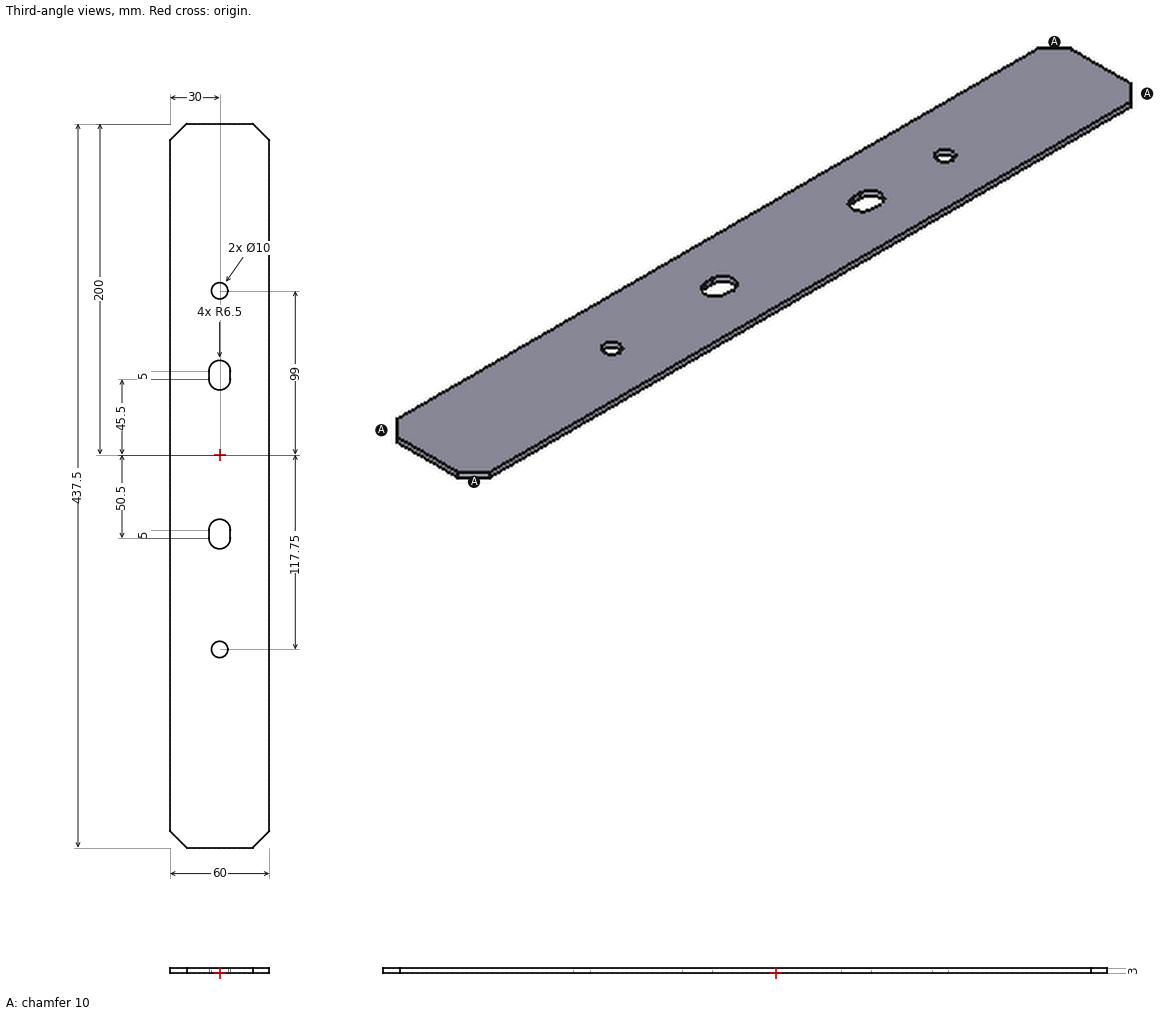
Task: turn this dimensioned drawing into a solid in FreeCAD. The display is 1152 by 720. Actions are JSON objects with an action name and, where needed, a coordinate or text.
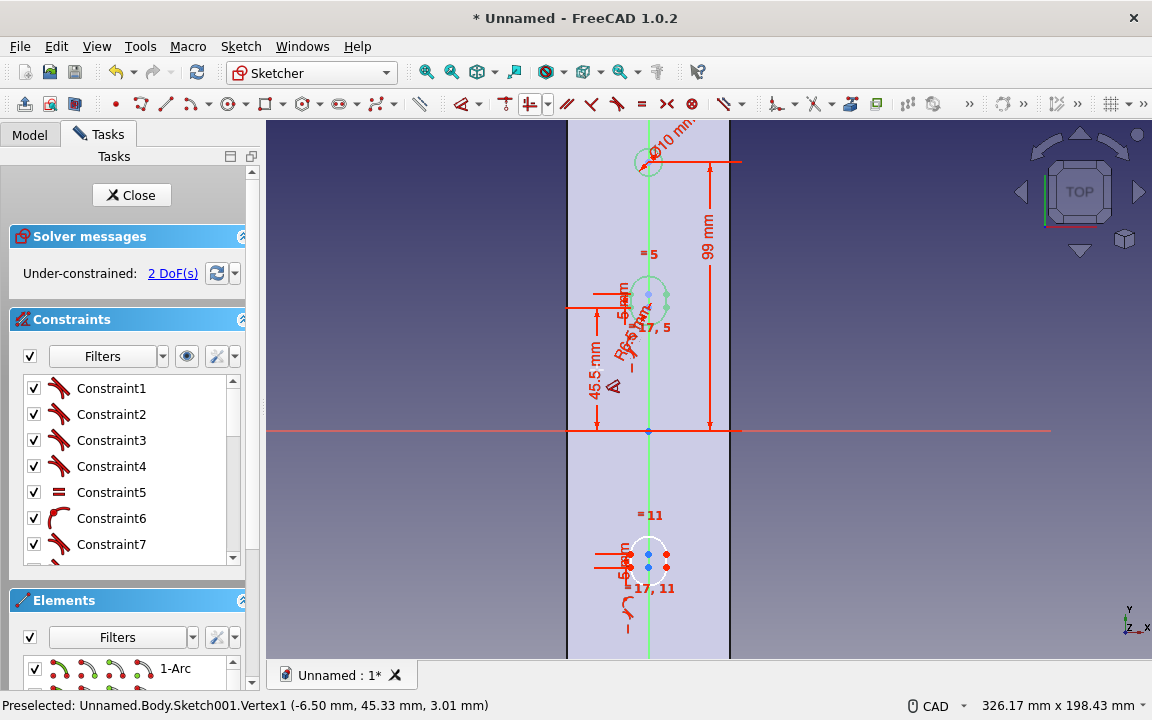
{"action": "left_click", "coordinate": [631, 568]}
{"action": "left_click", "coordinate": [597, 500]}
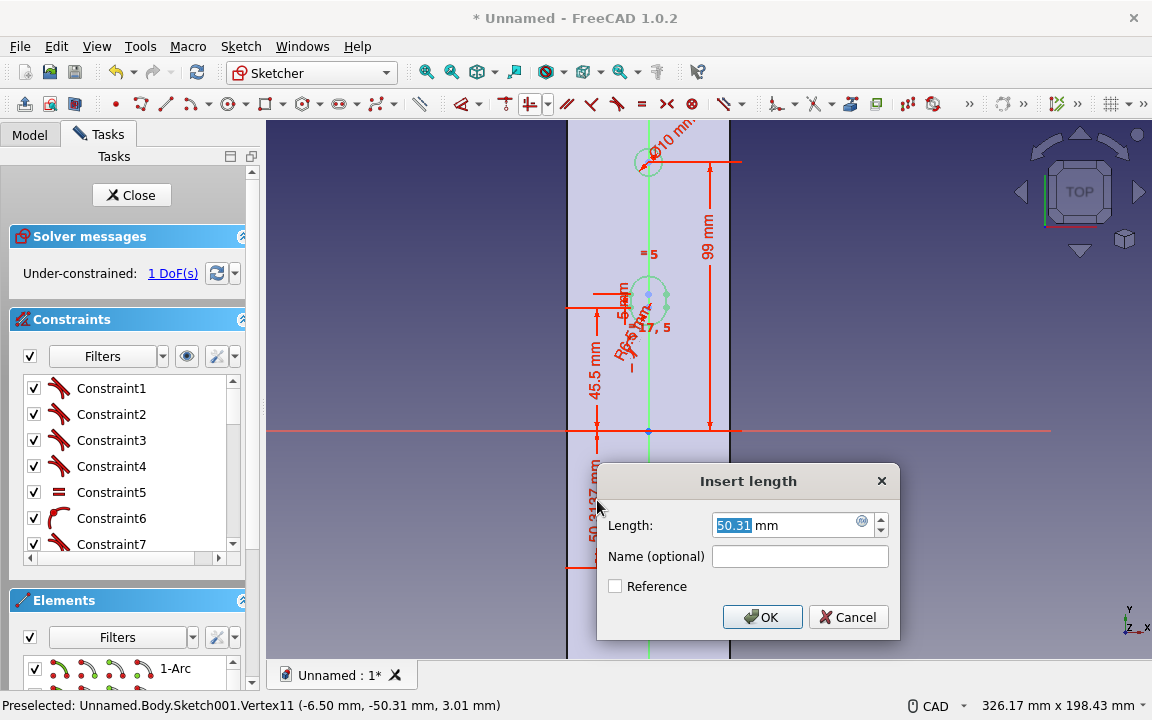
{"action": "type", "text": "50.5"}
{"action": "key", "text": "Return"}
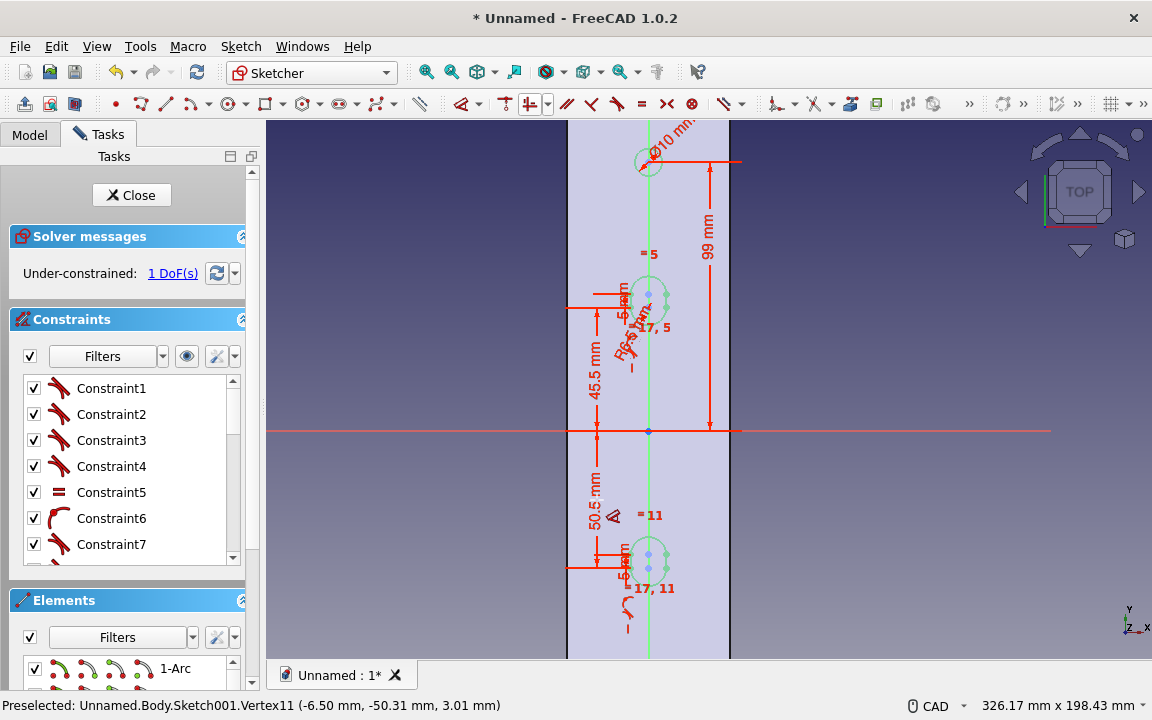
{"action": "scroll", "coordinate": [631, 308], "scroll_direction": "down", "scroll_amount": 3}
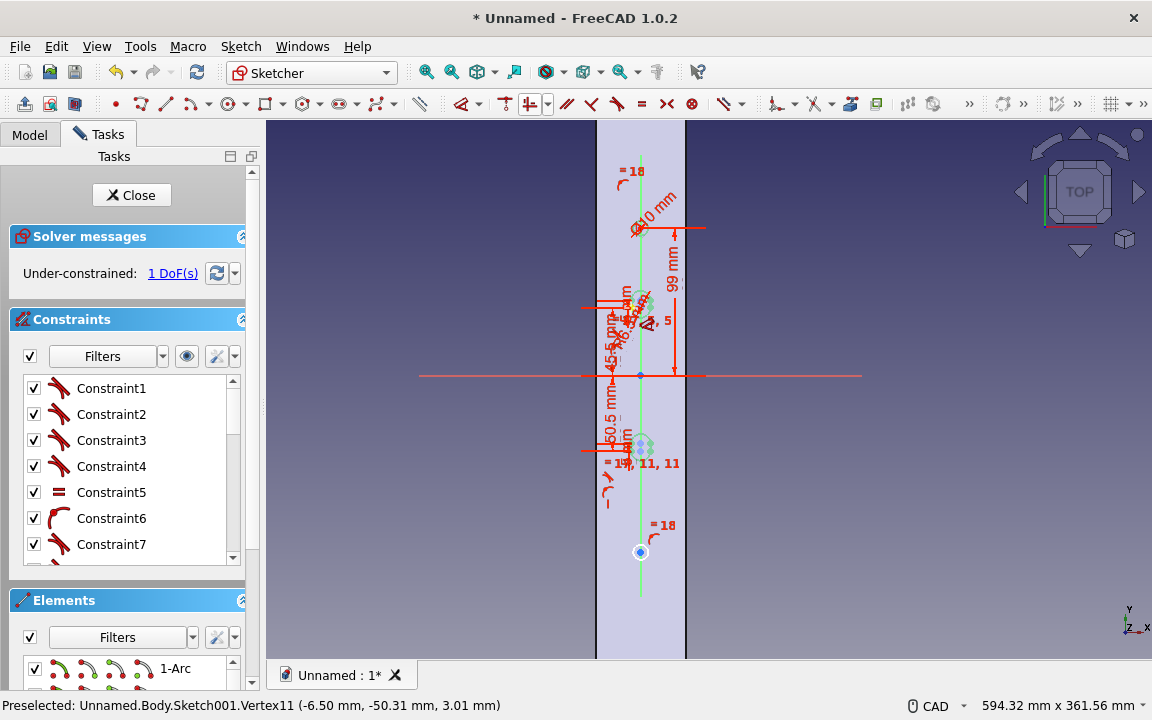
{"action": "left_click", "coordinate": [641, 552]}
{"action": "left_click", "coordinate": [675, 505]}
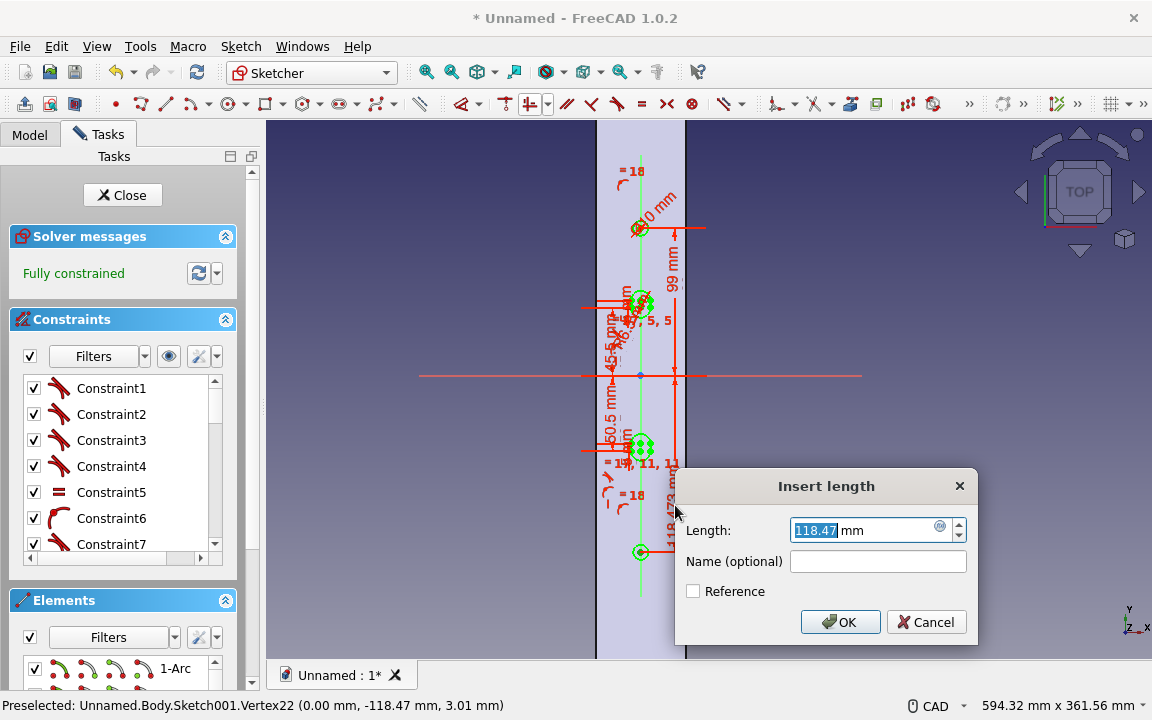
{"action": "type", "text": "117.75"}
{"action": "key", "text": "Return"}
{"action": "key", "text": "Escape"}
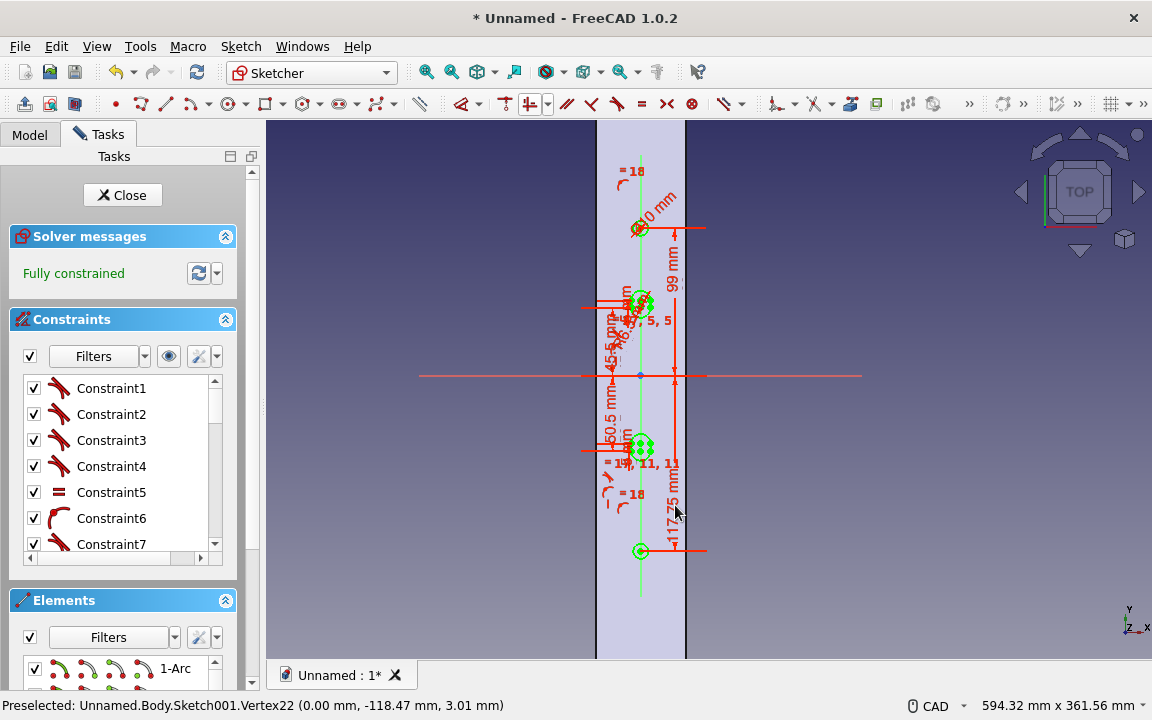
{"action": "left_click", "coordinate": [123, 195]}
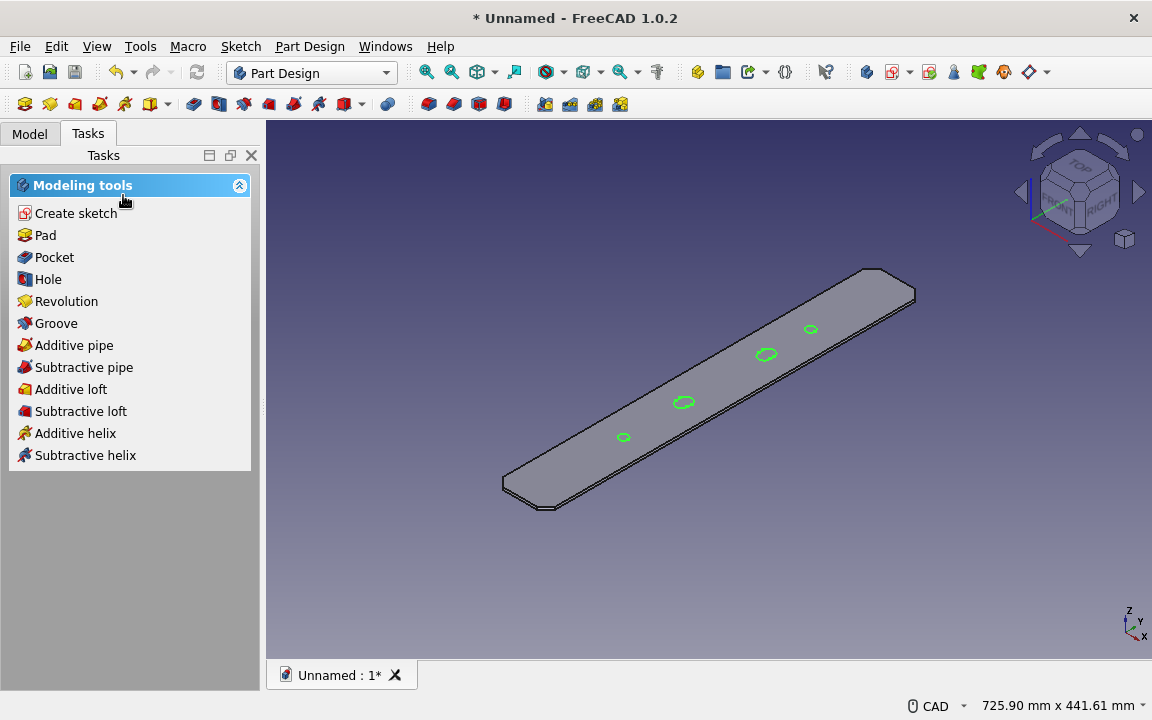
{"action": "left_click", "coordinate": [194, 104]}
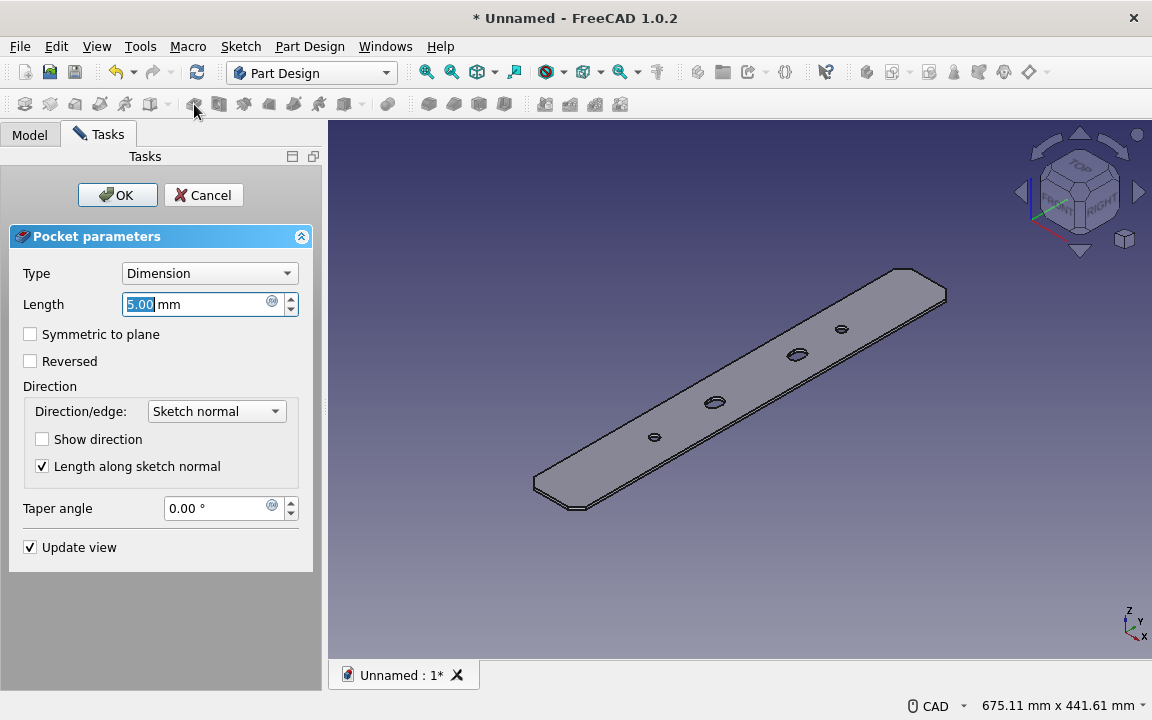
{"action": "type", "text": "10"}
{"action": "key", "text": "Tab"}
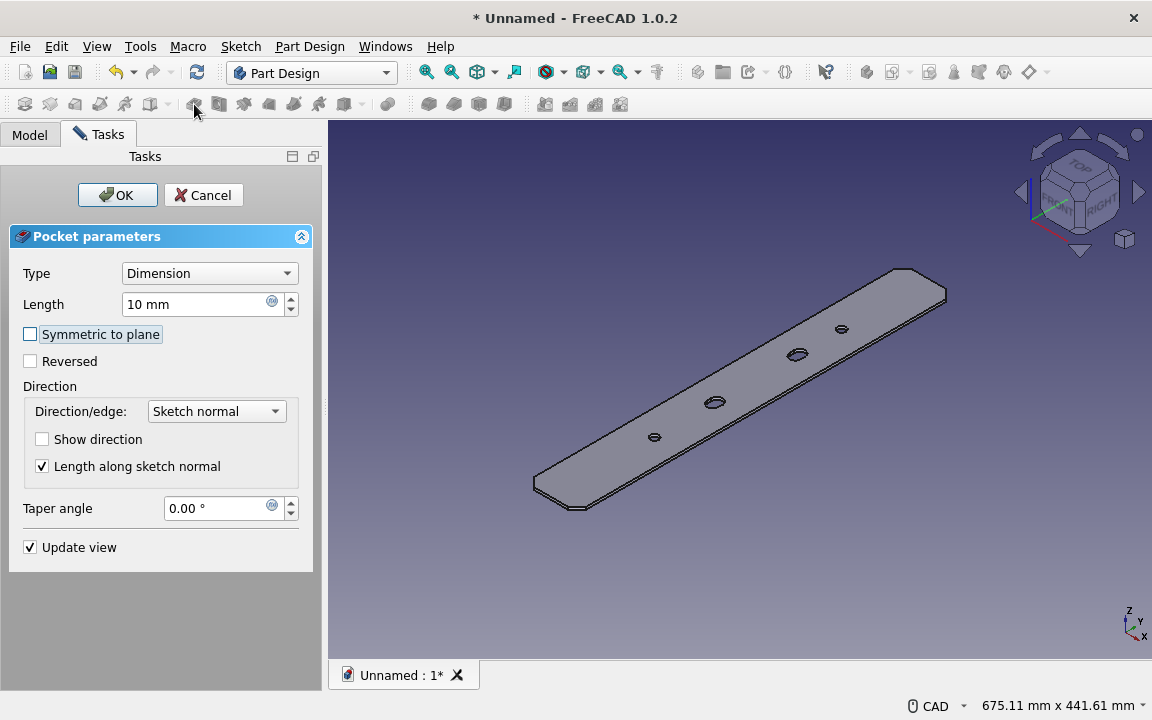
{"action": "left_click", "coordinate": [118, 195]}